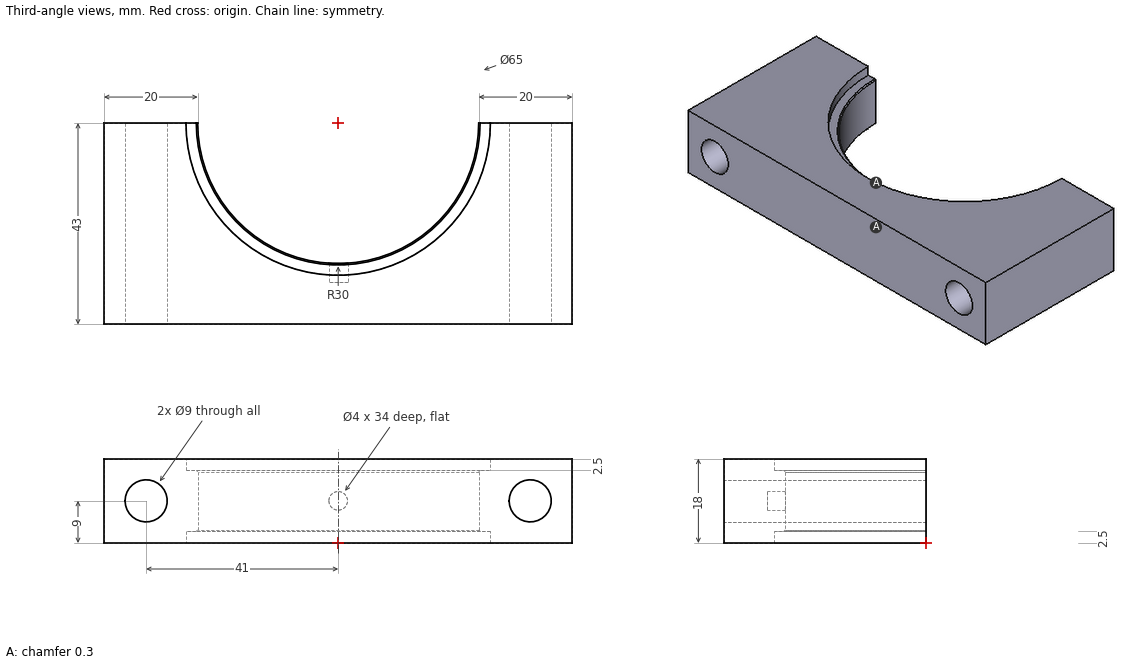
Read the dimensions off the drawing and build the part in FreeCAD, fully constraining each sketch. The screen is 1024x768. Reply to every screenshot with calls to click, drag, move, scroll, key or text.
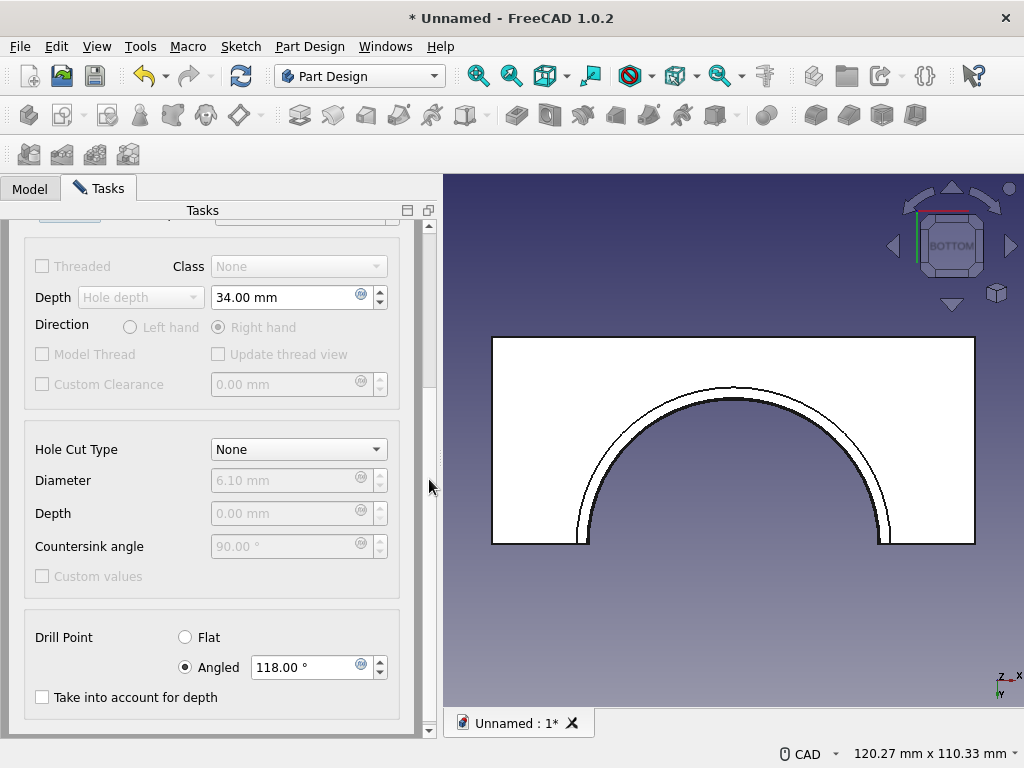
click(186, 635)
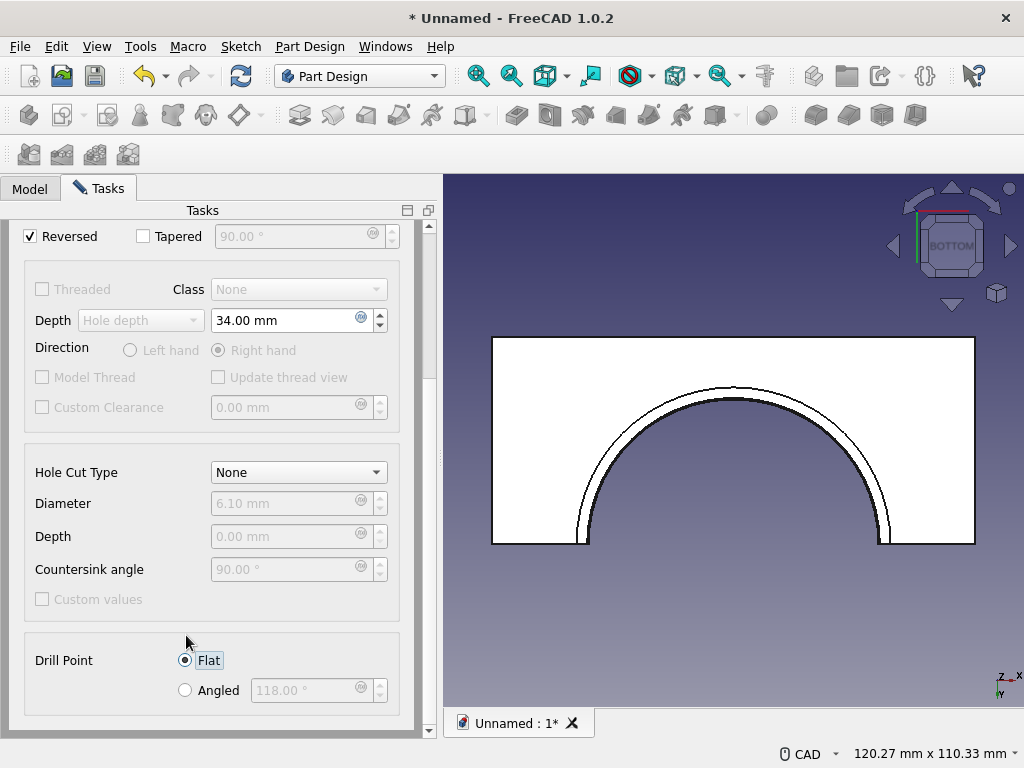
scroll(429, 479, up, 5)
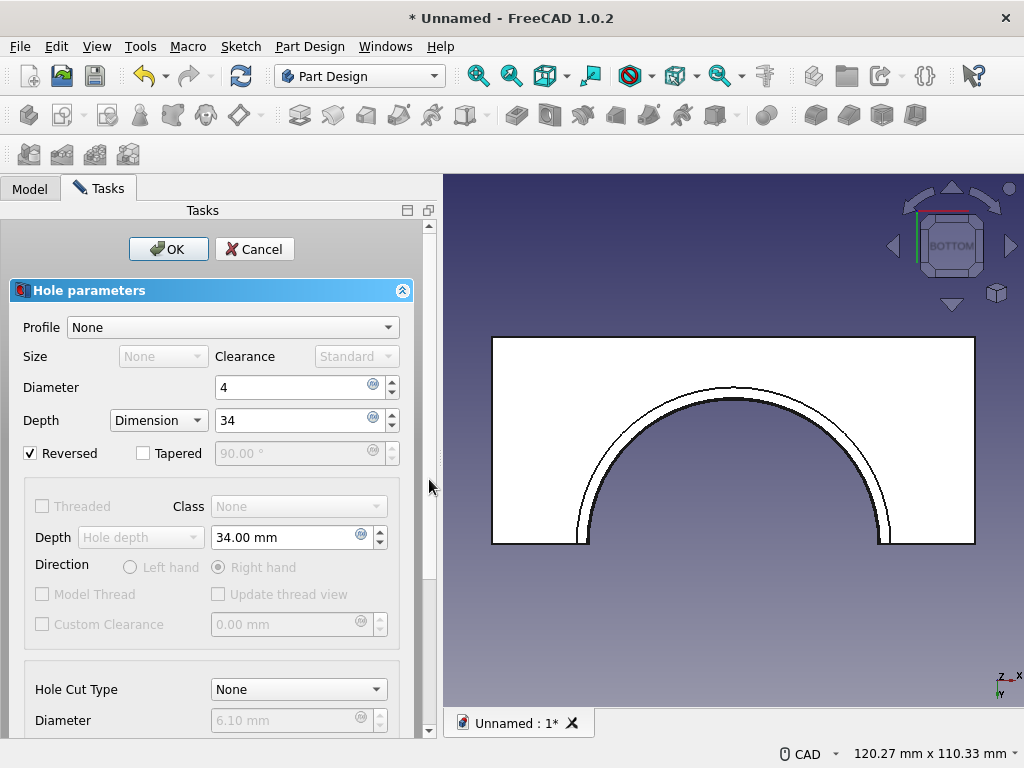
click(169, 249)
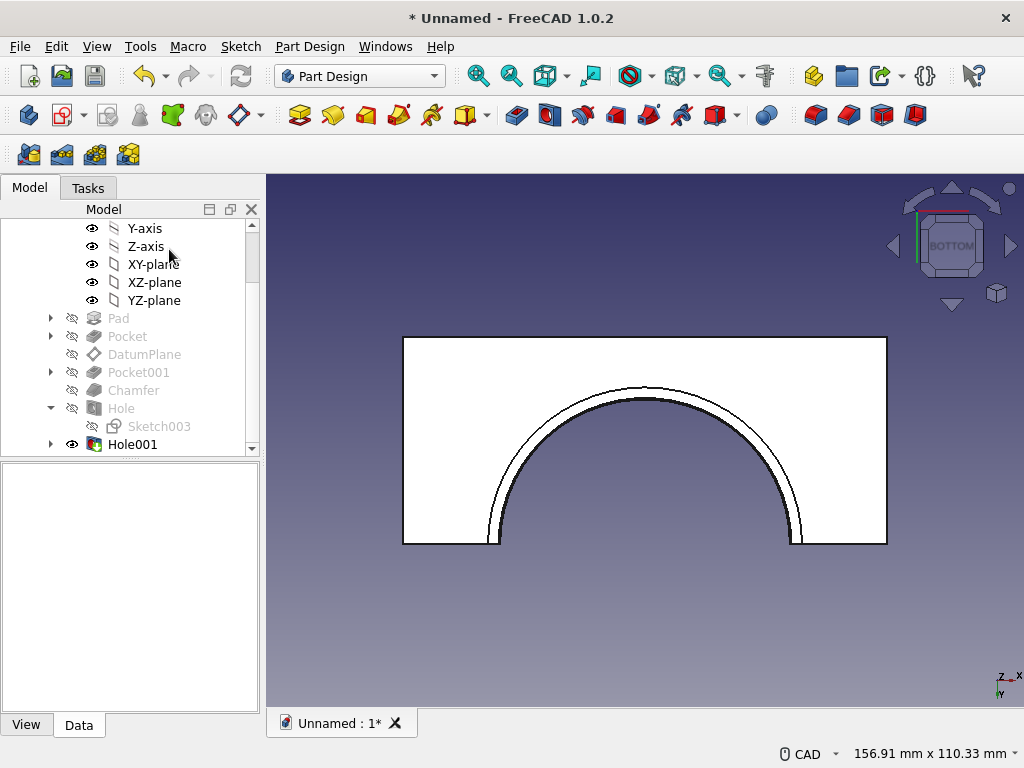
key(0)